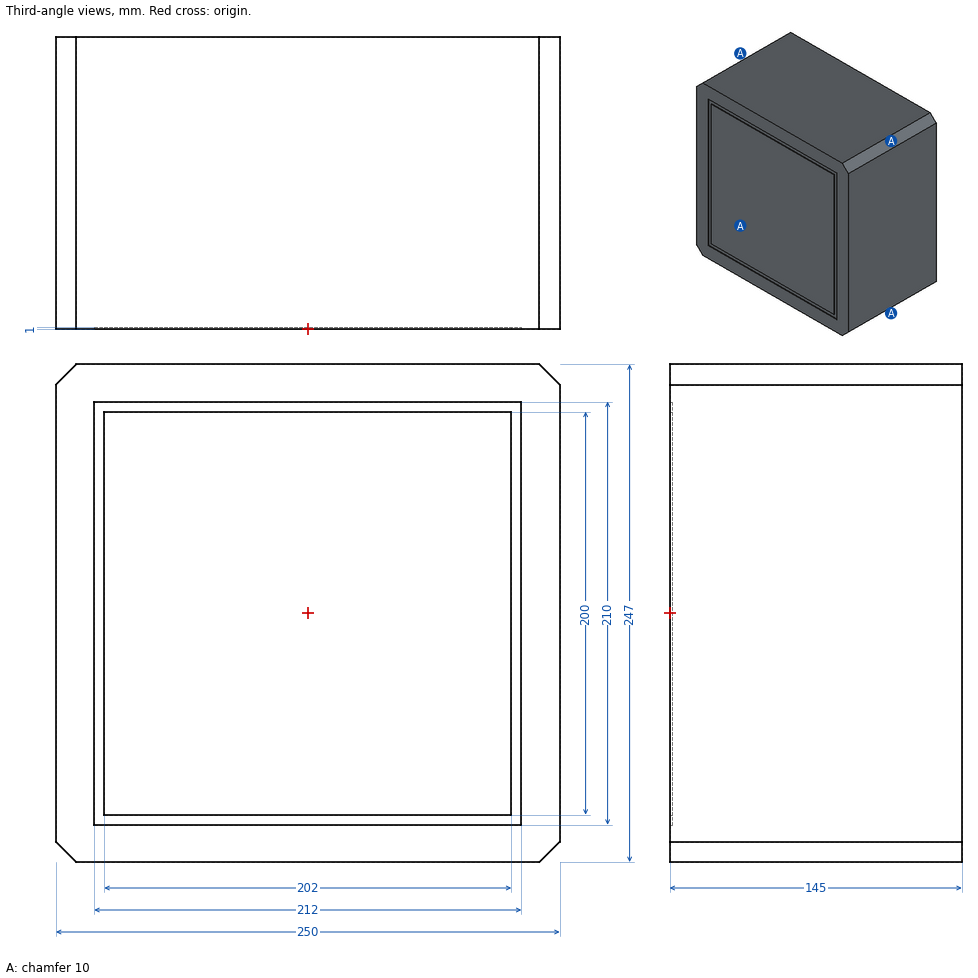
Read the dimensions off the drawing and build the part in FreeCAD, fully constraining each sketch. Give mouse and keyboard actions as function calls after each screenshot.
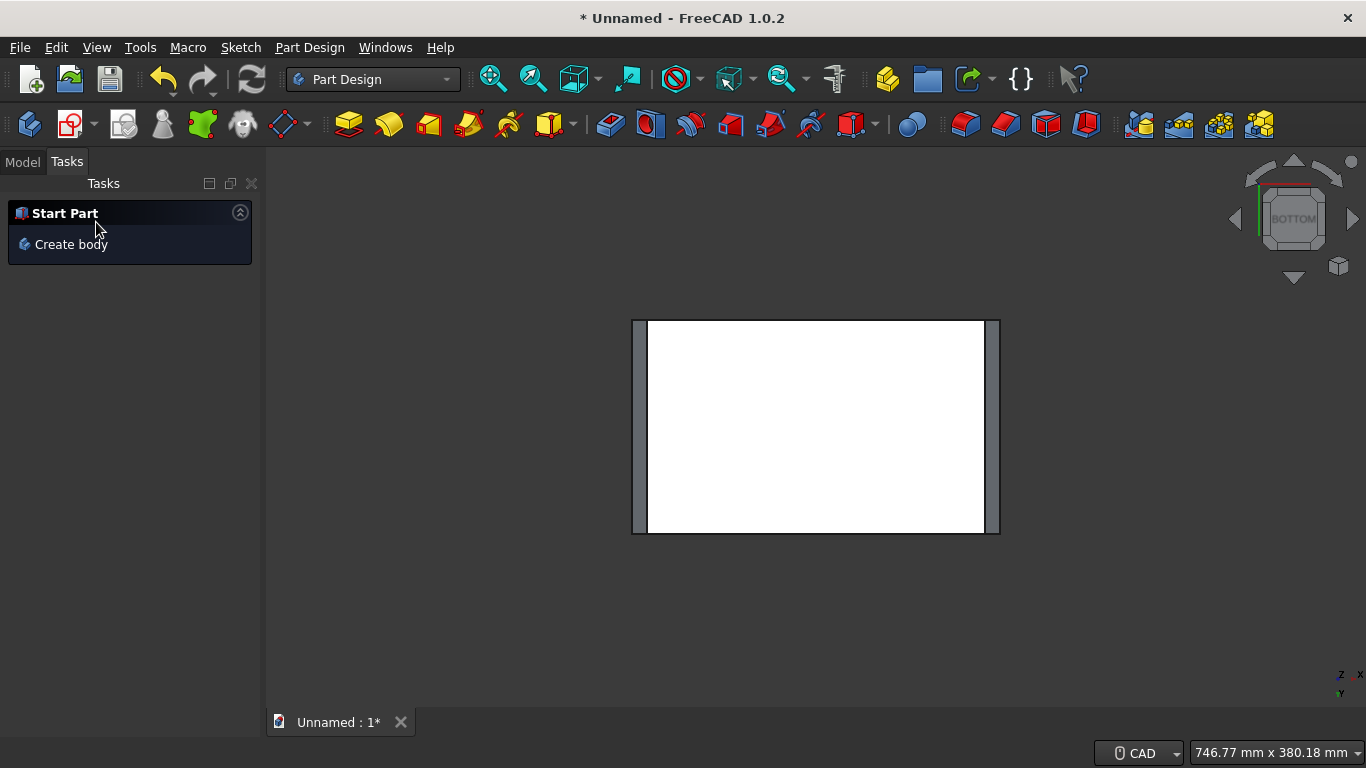
key(0)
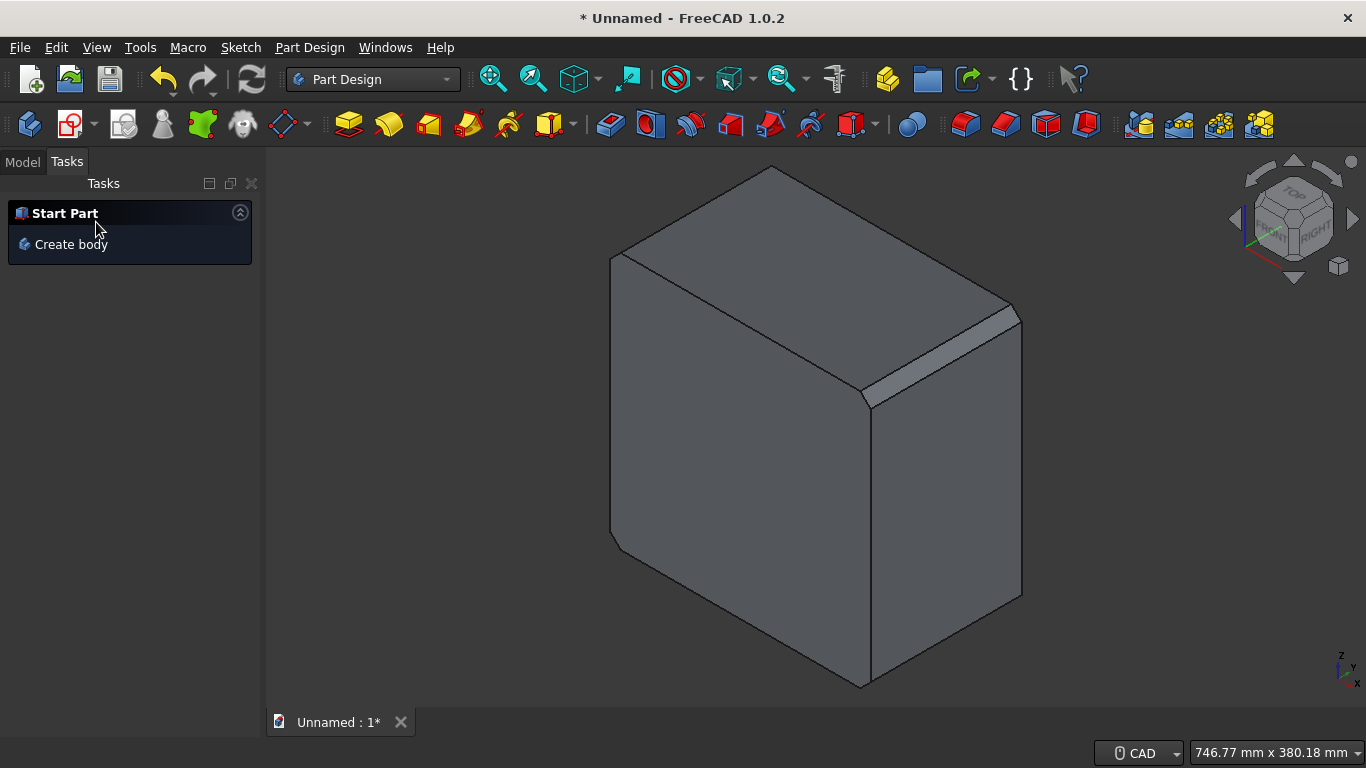
click(740, 470)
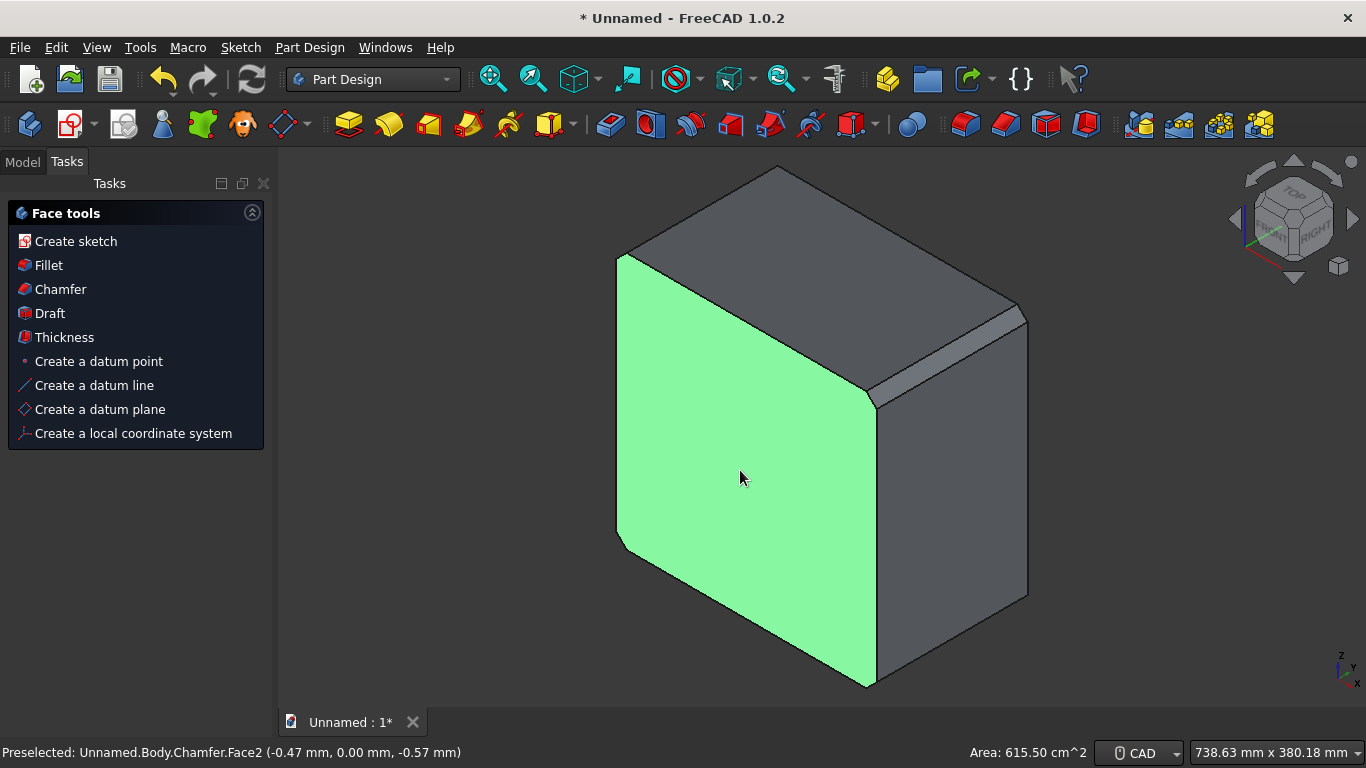
click(70, 124)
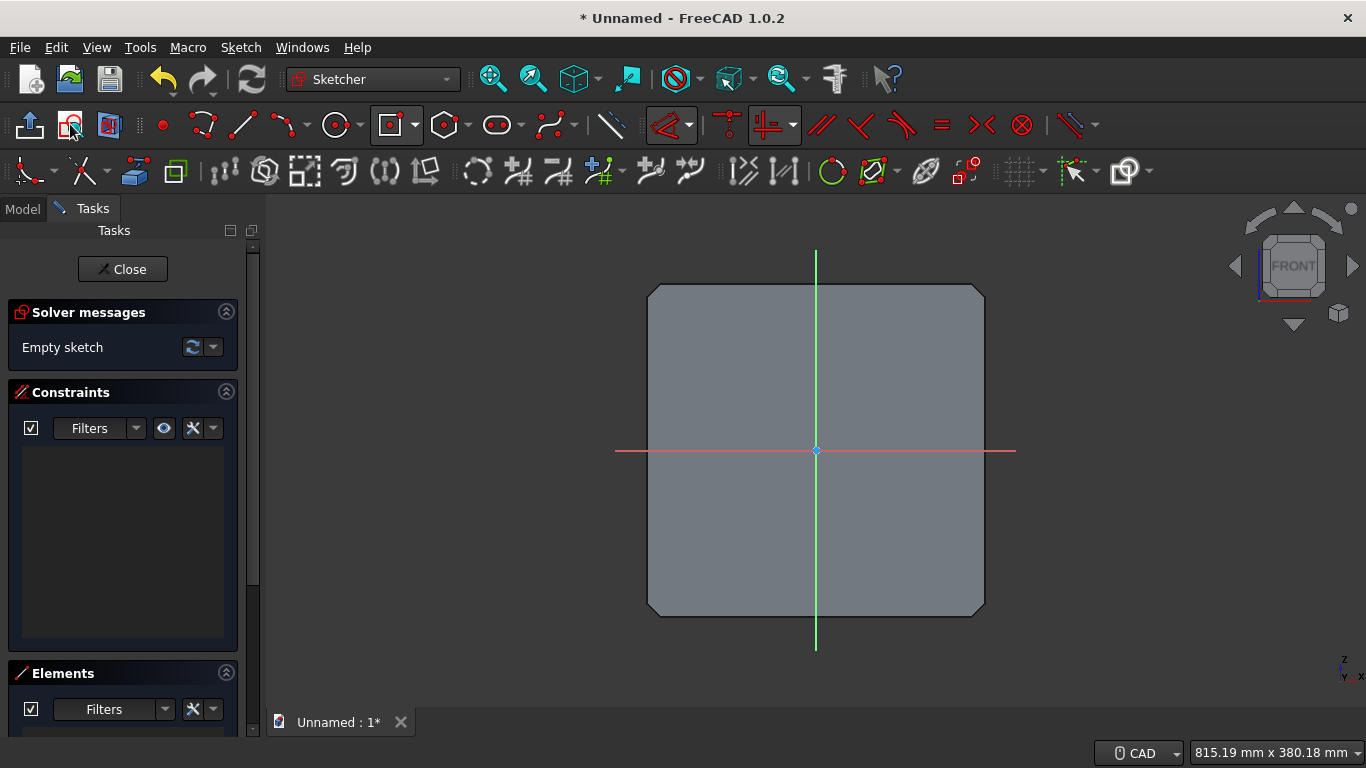
key(g)
key(v)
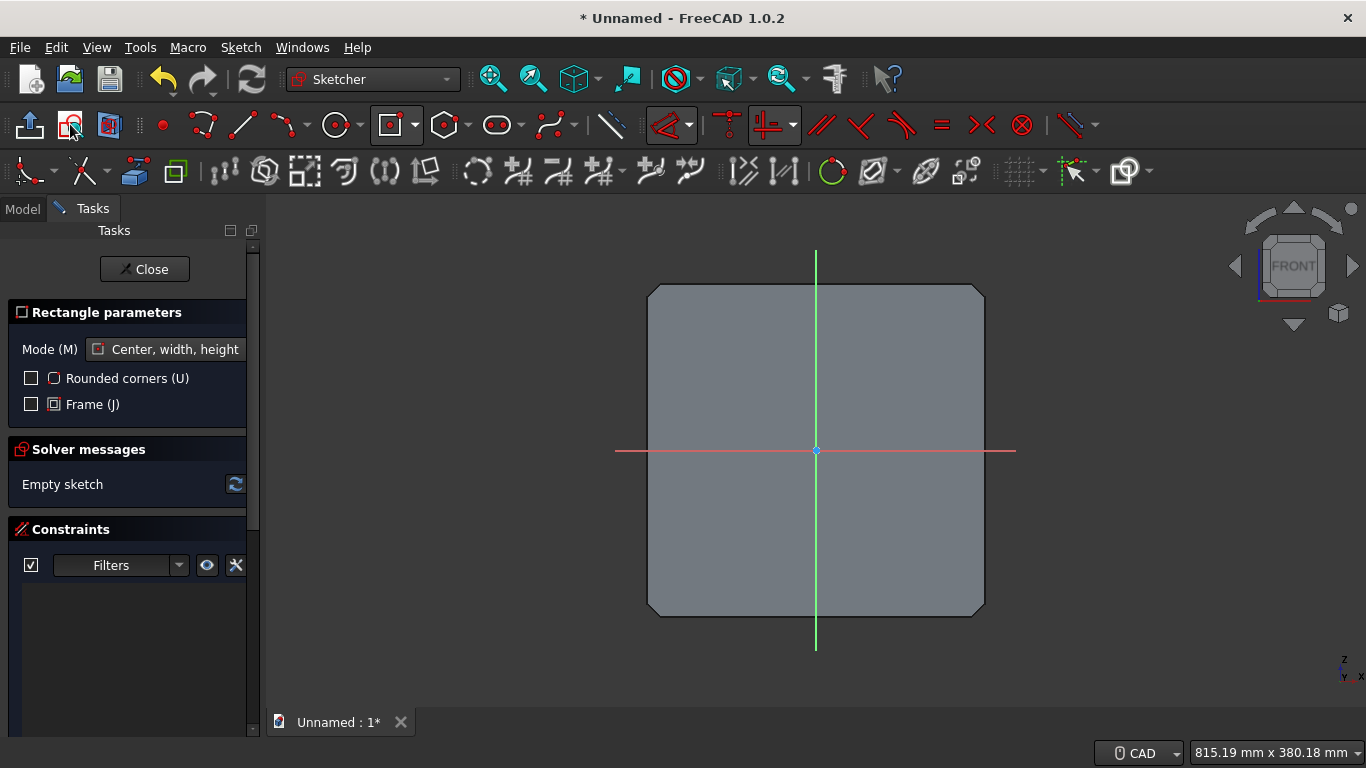
click(816, 450)
move(959, 309)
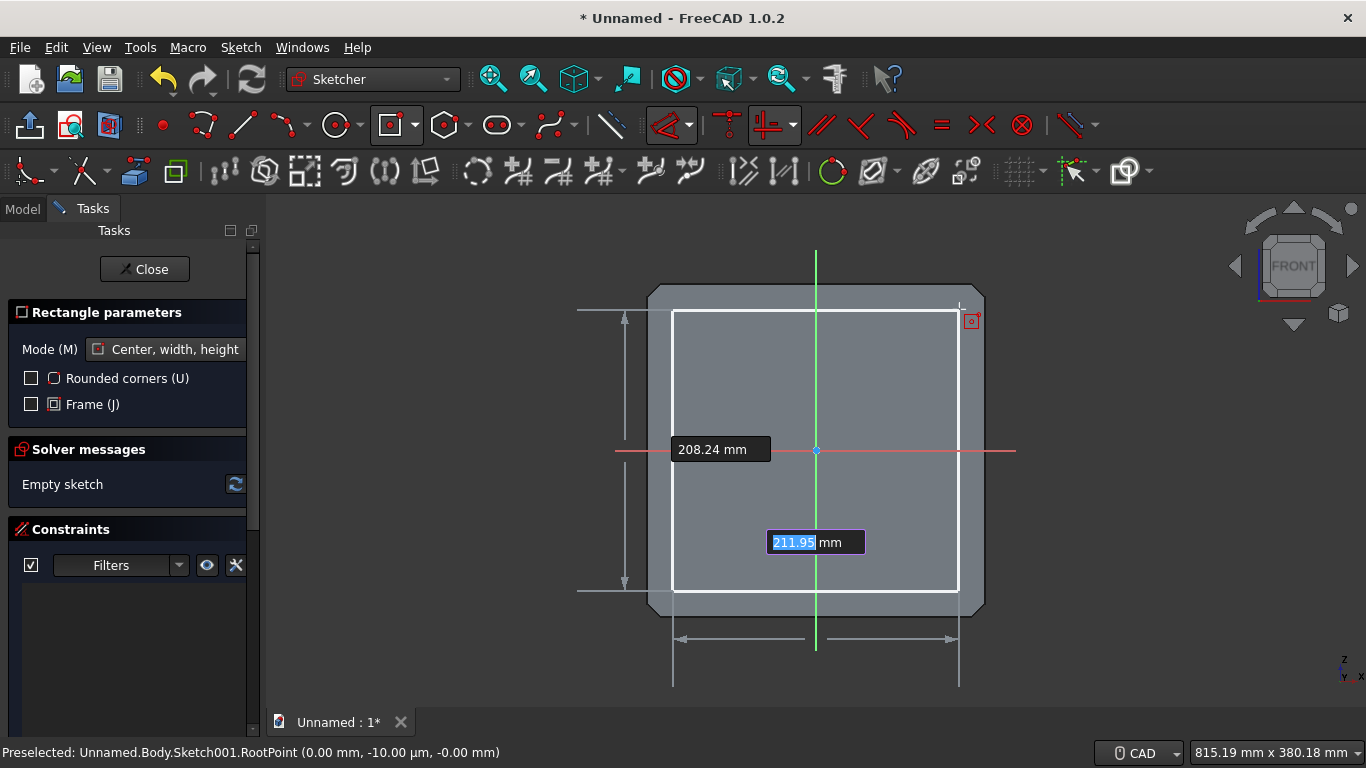
text(212)
key(Tab)
text(210)
key(Return)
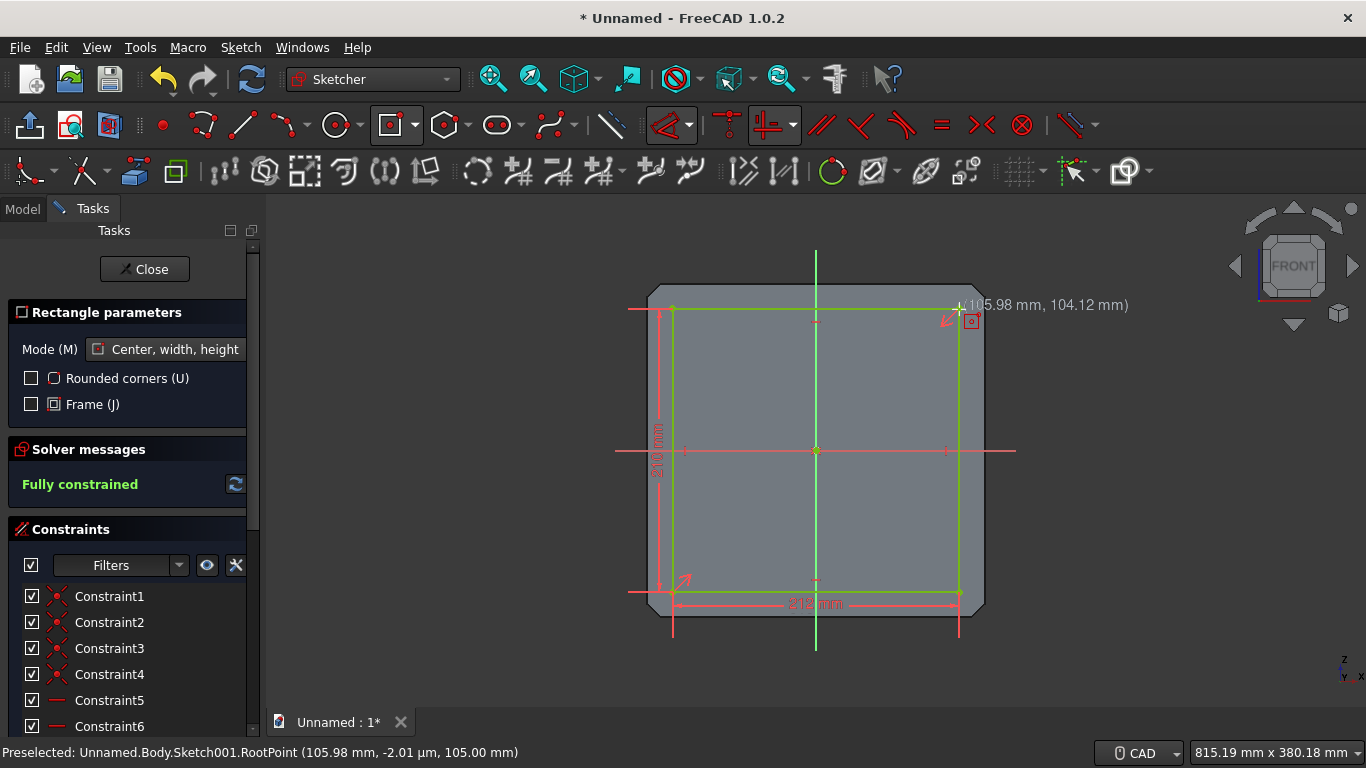
click(816, 450)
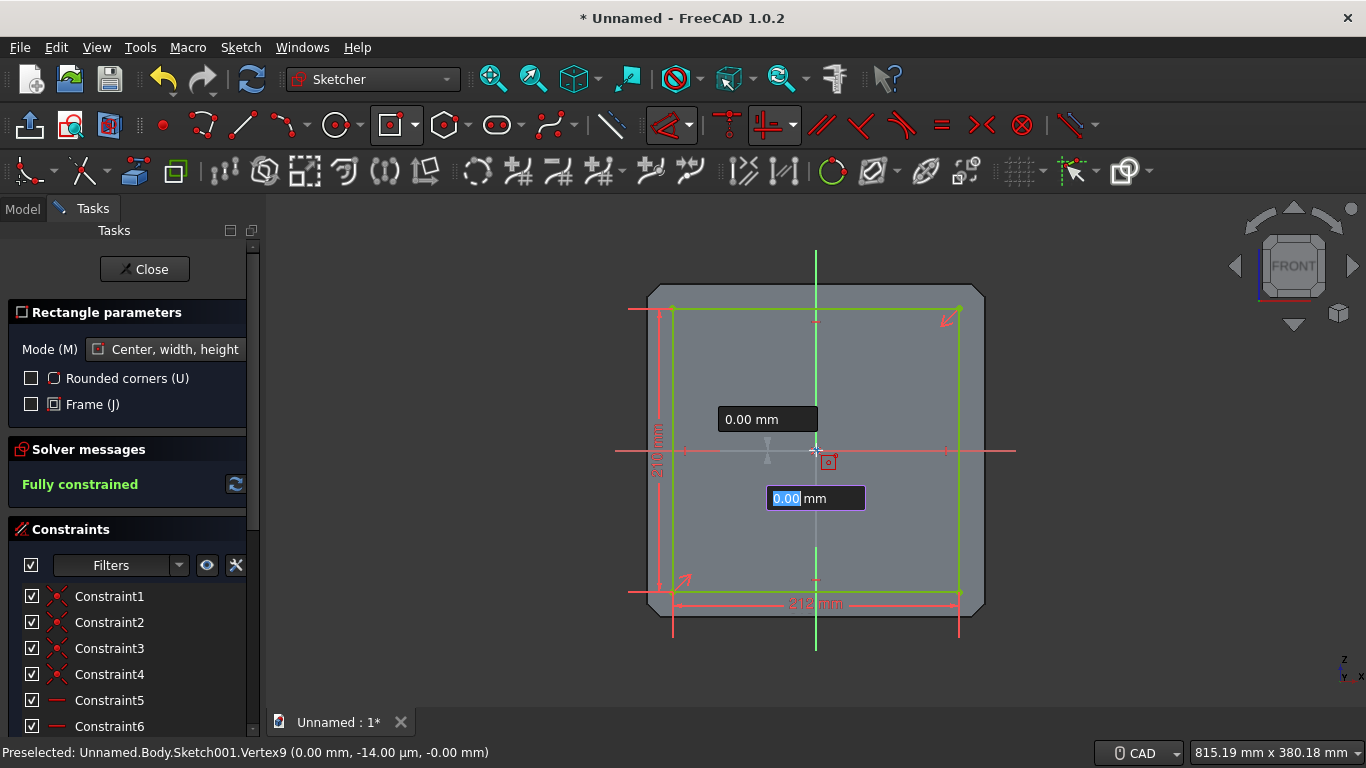
scroll(952, 316, up, 5)
move(952, 314)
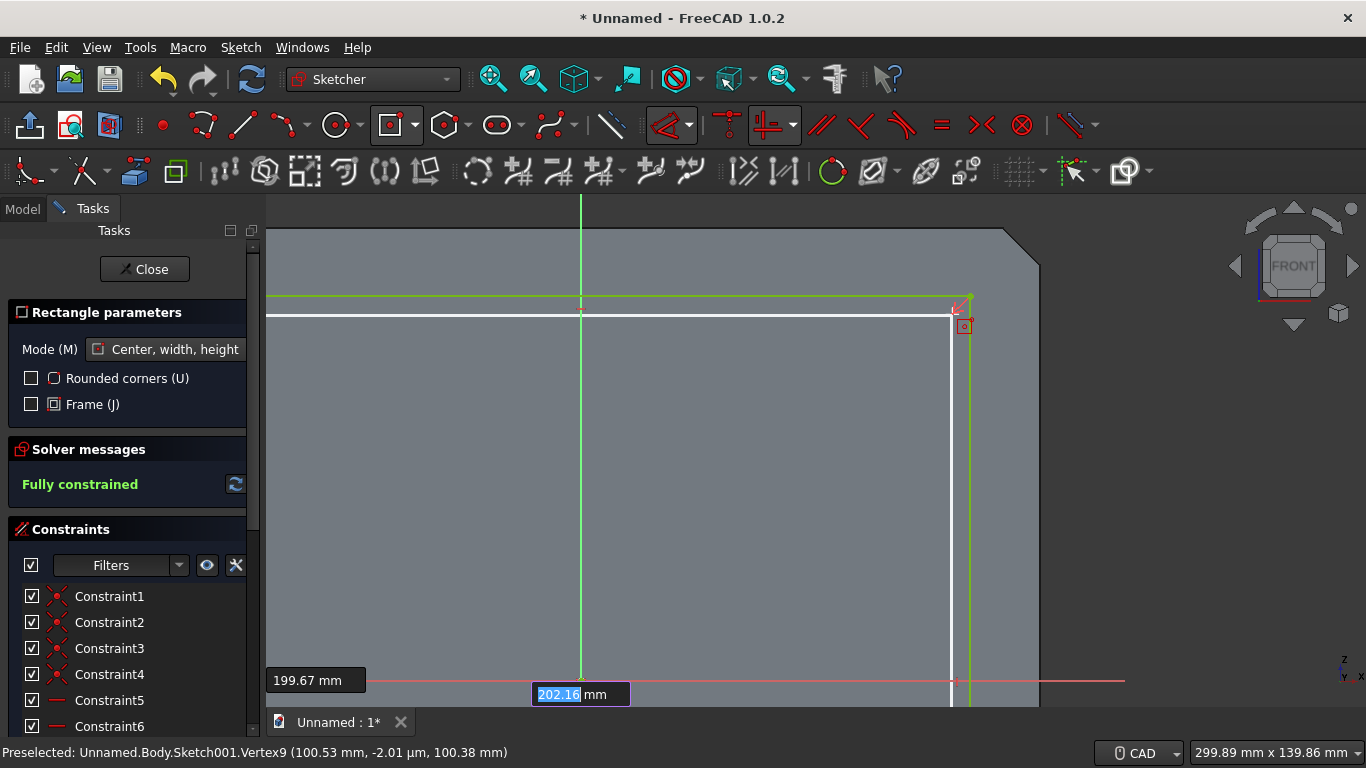
text(202)
key(Tab)
text(200)
key(Return)
key(Escape)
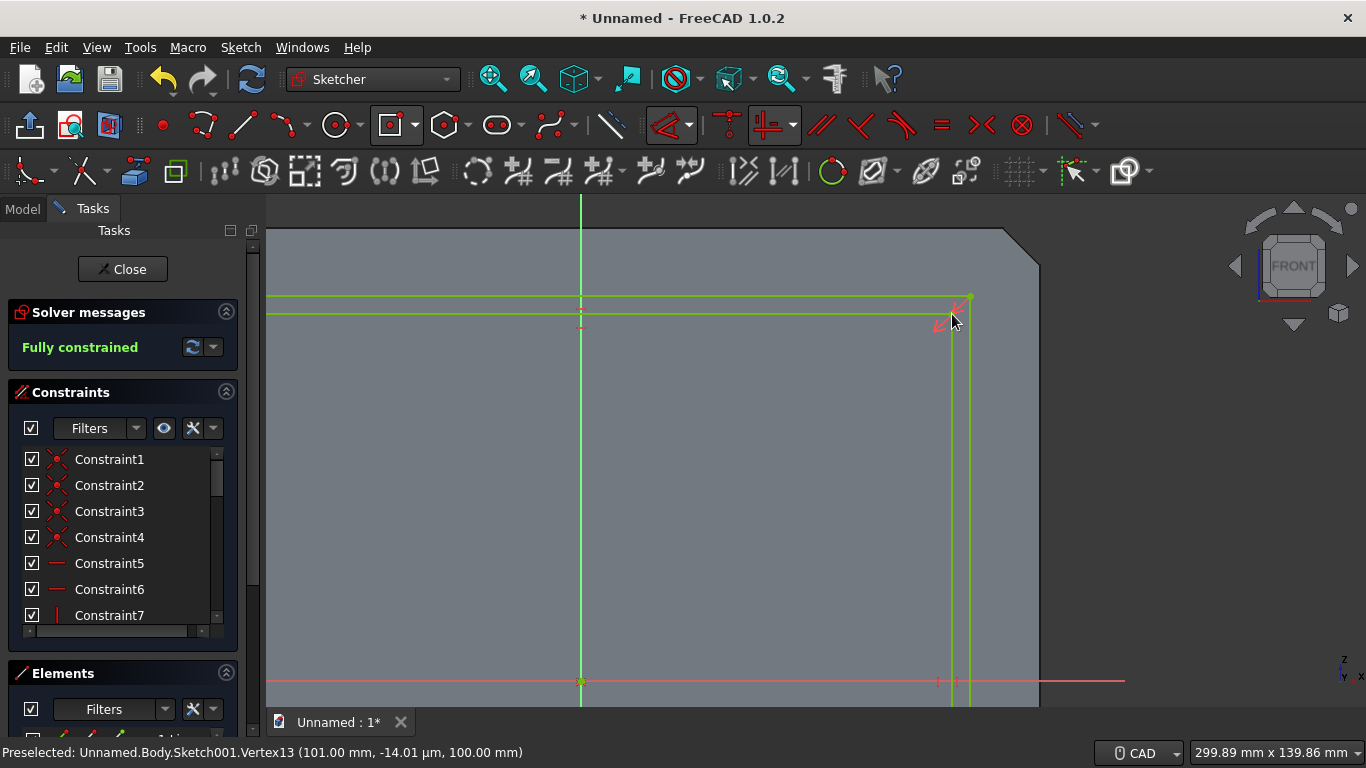
click(123, 269)